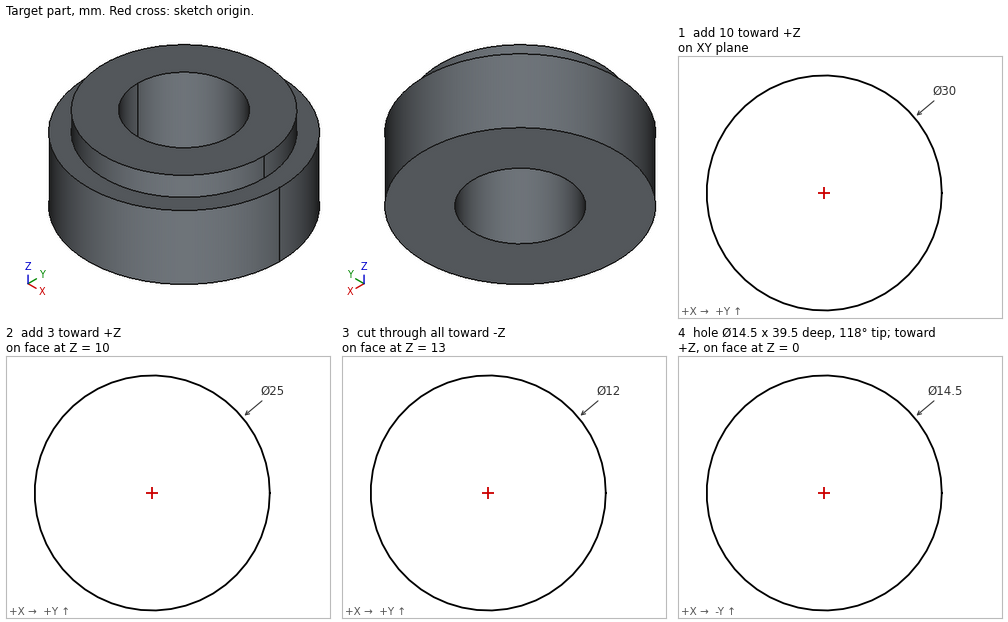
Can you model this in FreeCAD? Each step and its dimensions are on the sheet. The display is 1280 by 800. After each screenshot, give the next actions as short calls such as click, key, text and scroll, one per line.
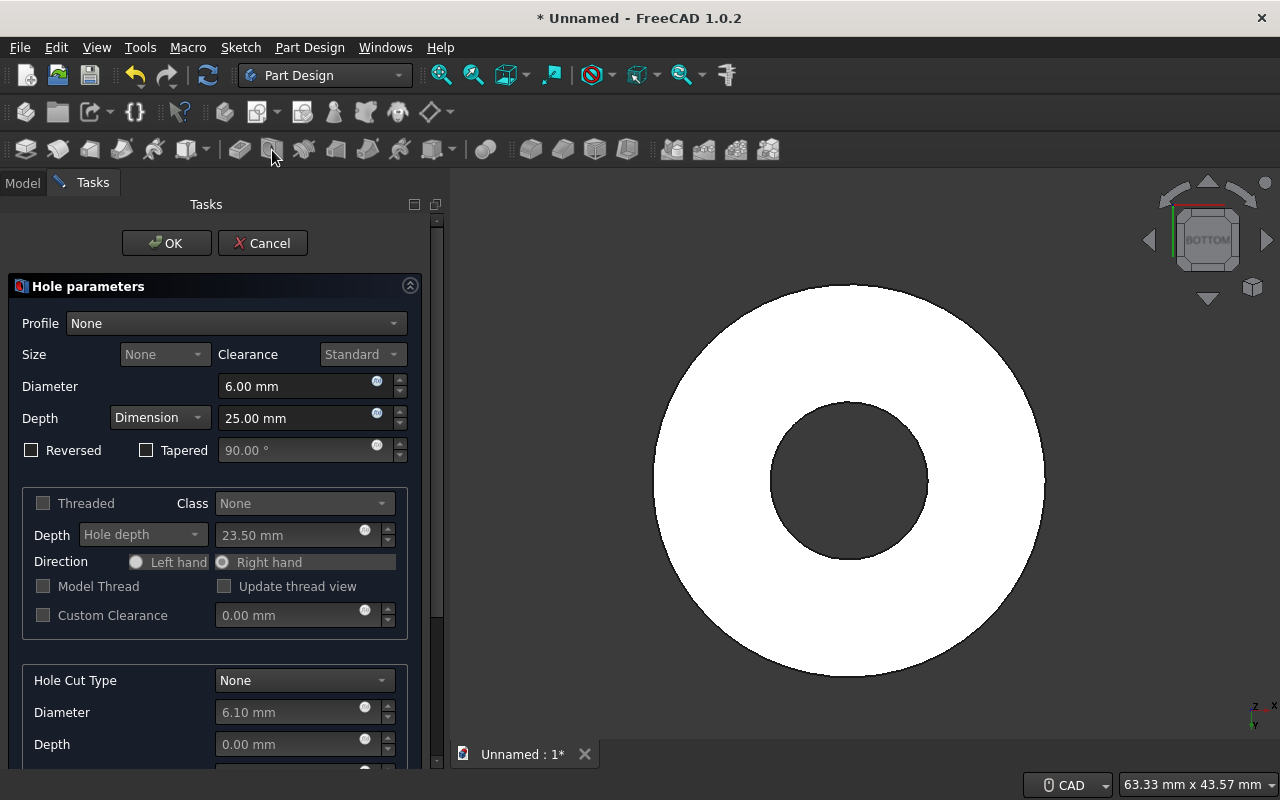
triple_click(305, 386)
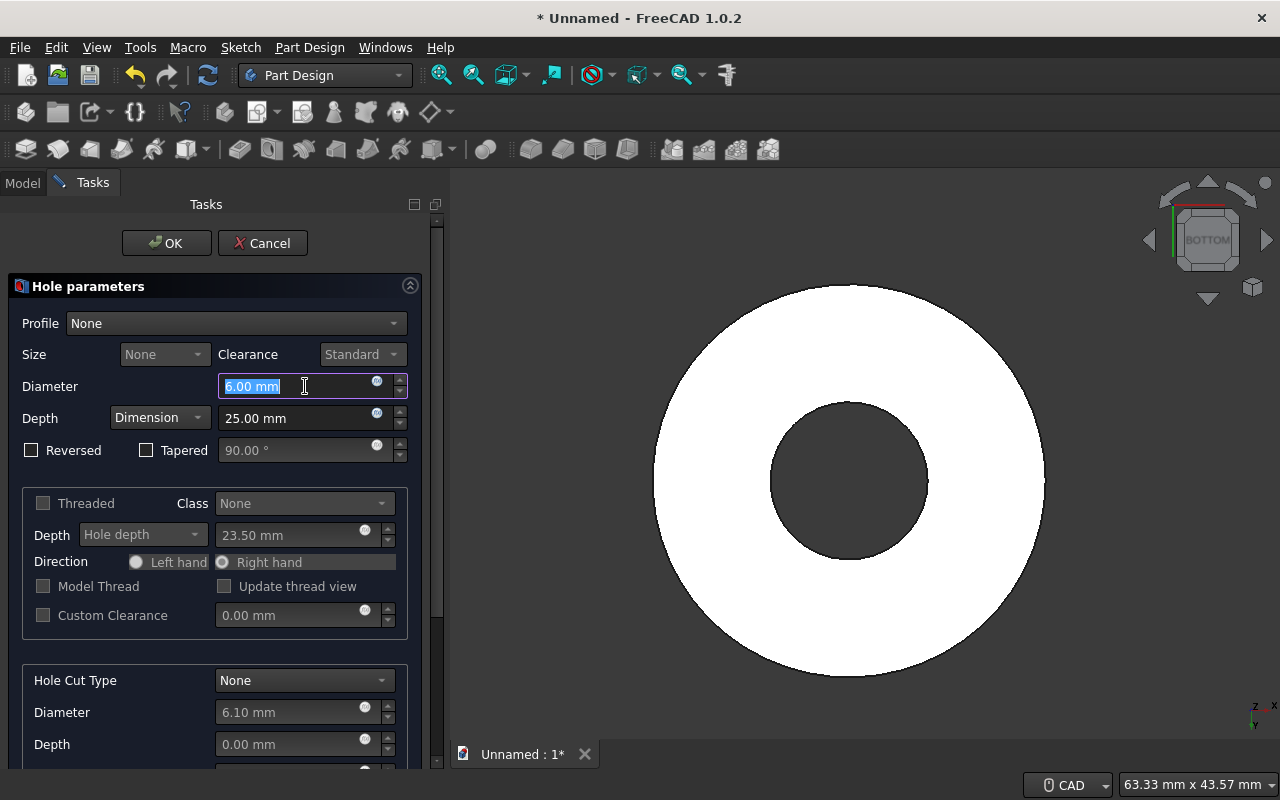
text(14.5)
key(Tab)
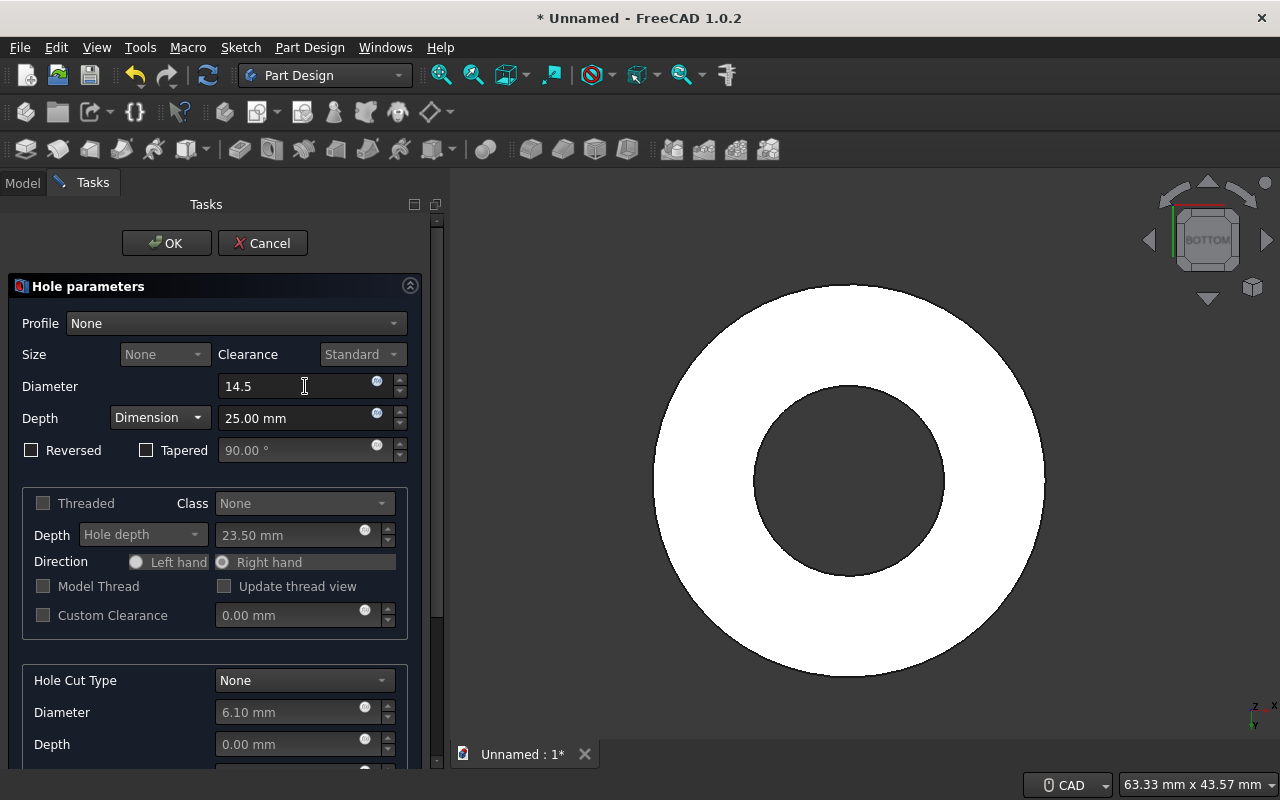
triple_click(305, 418)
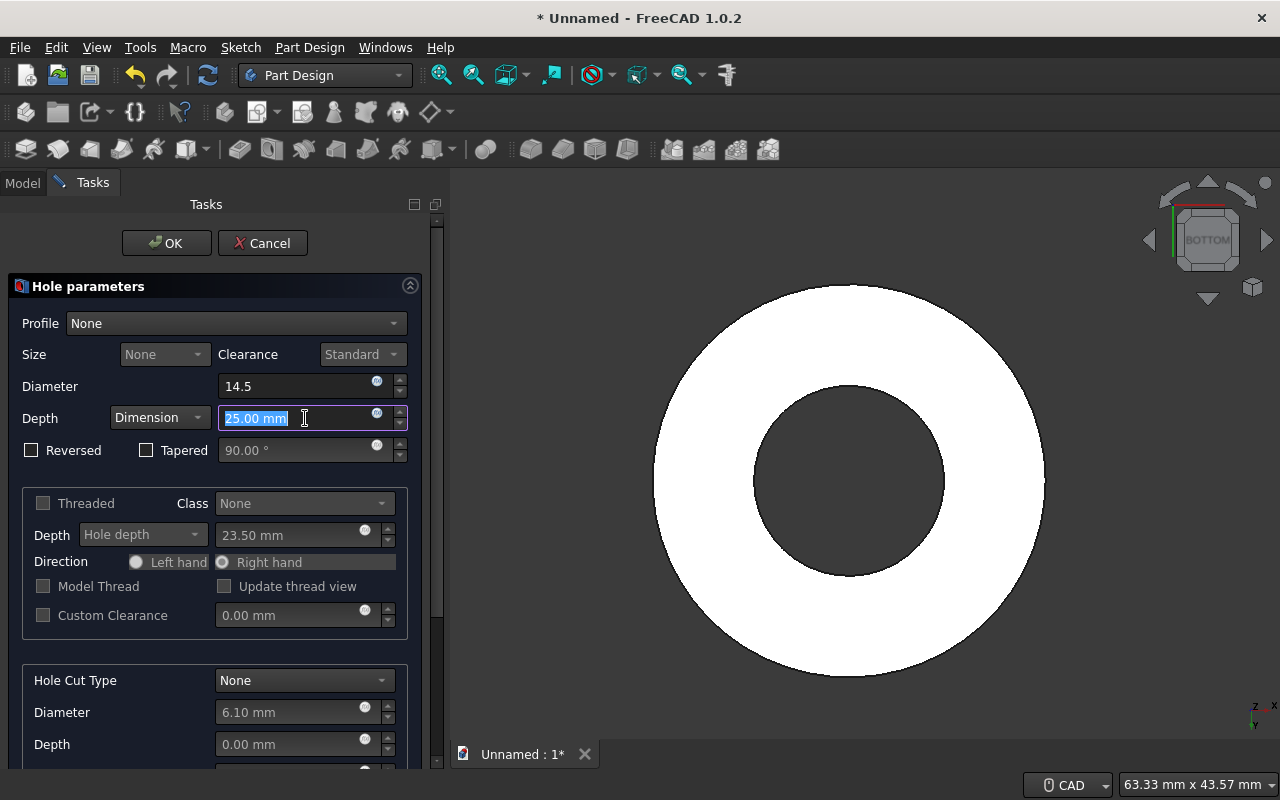
text(39.5)
key(Tab)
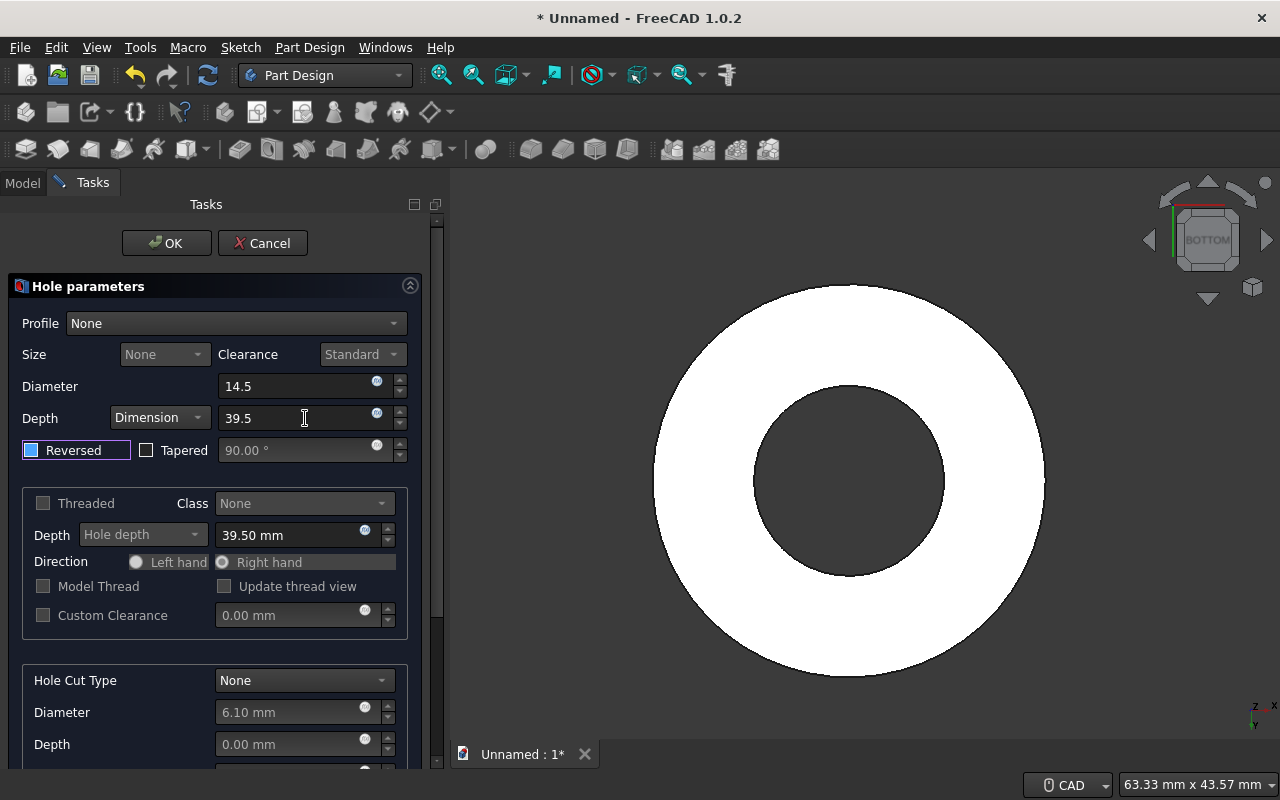
click(167, 243)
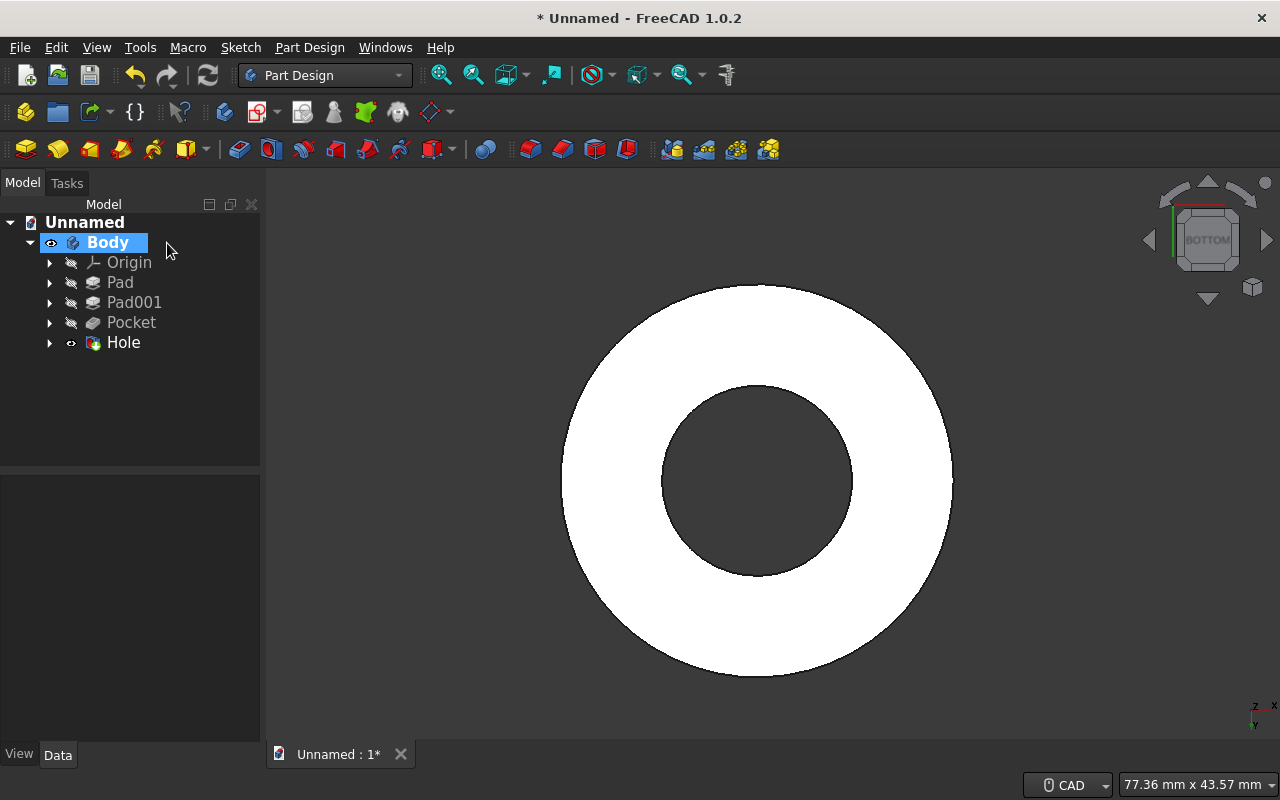
key(0)